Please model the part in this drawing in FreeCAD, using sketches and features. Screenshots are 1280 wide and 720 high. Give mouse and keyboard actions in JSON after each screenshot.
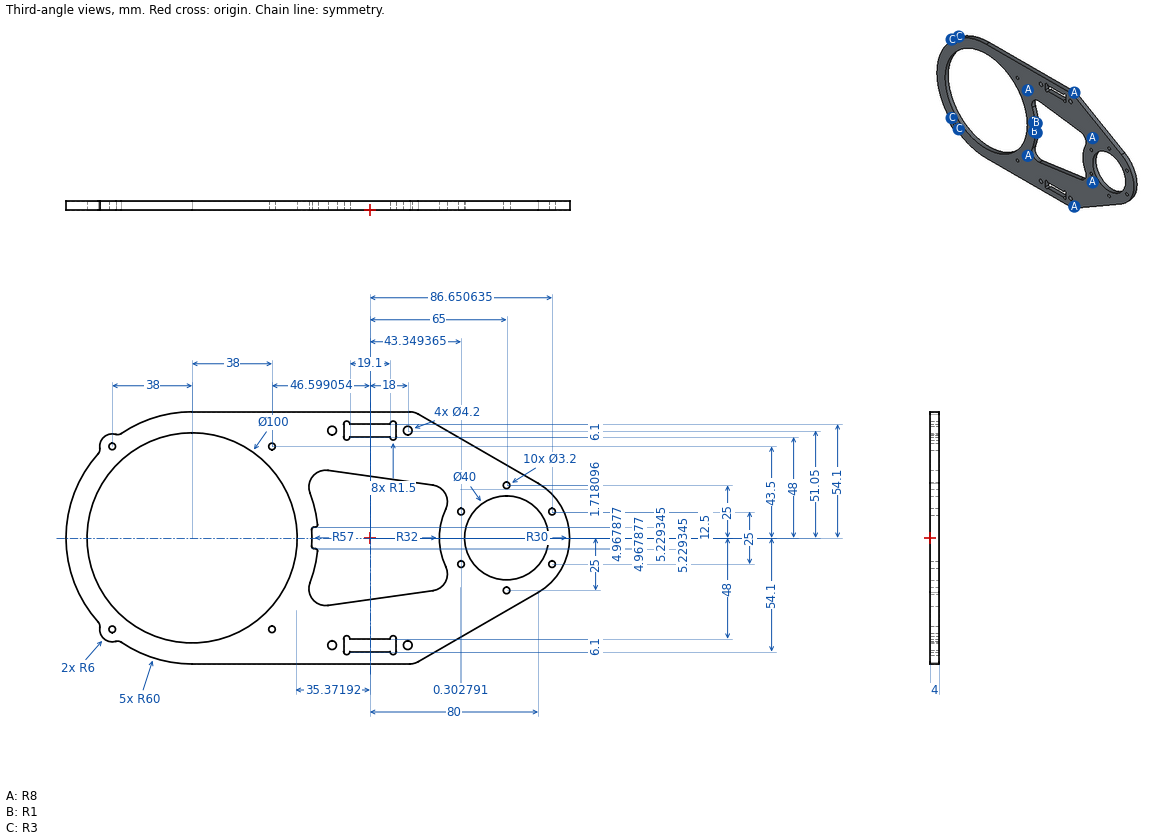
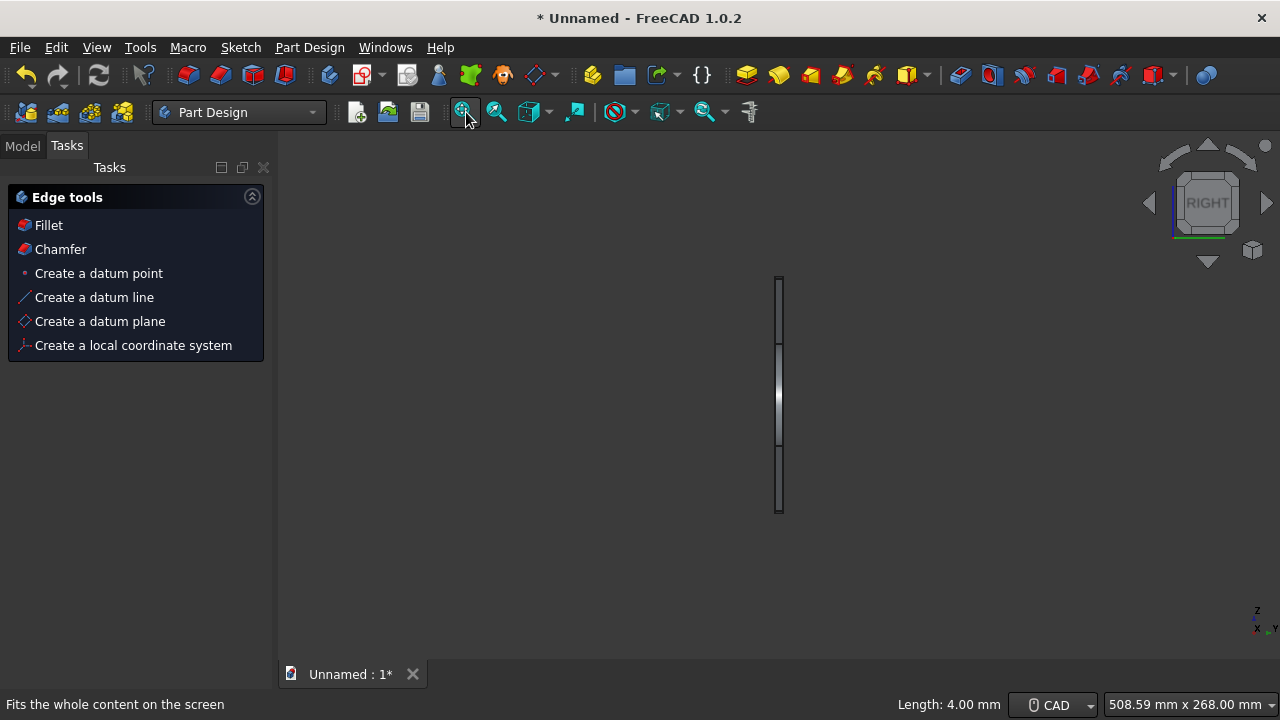
{"action": "key", "text": "5"}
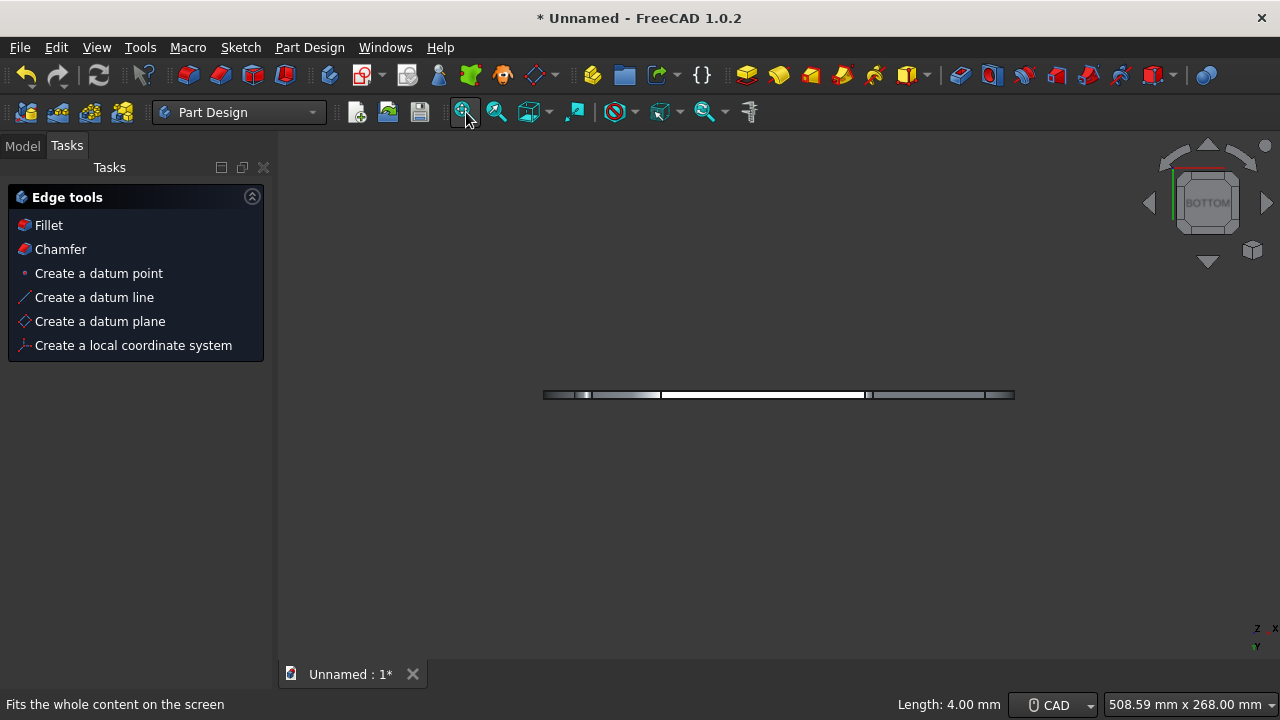
{"action": "scroll", "coordinate": [773, 394], "scroll_direction": "up", "scroll_amount": 9}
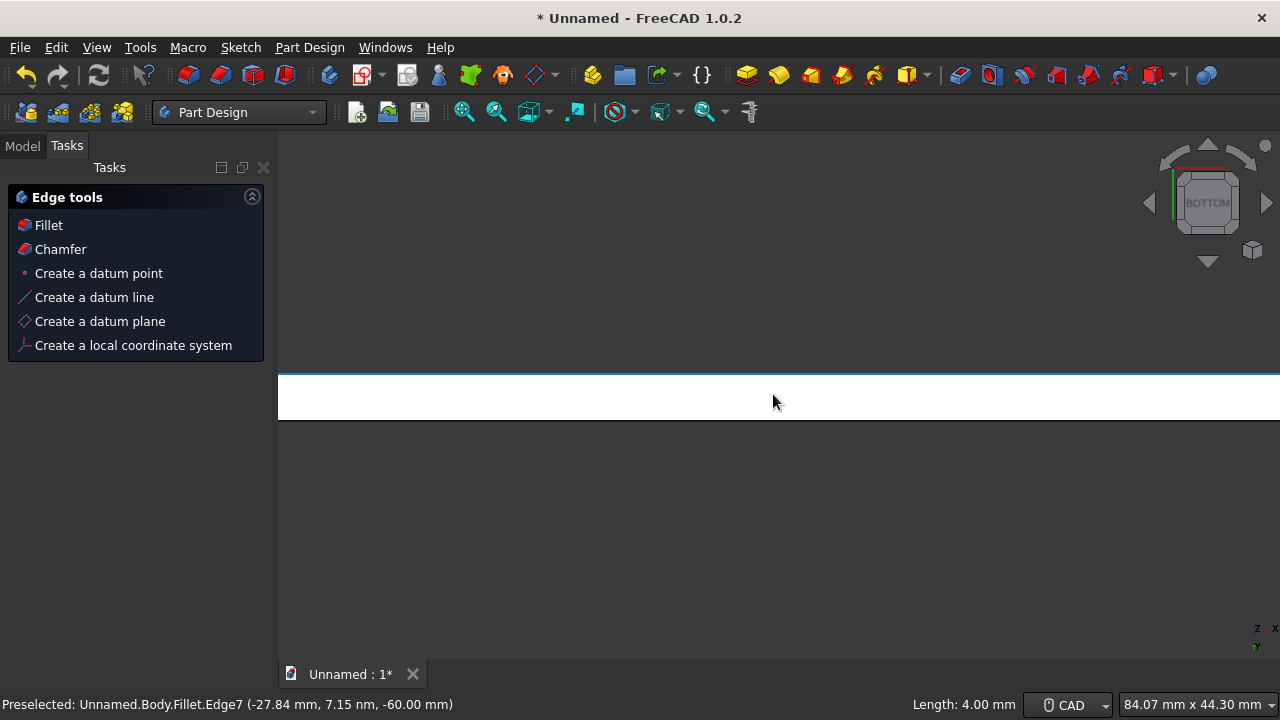
{"action": "left_click", "coordinate": [466, 112]}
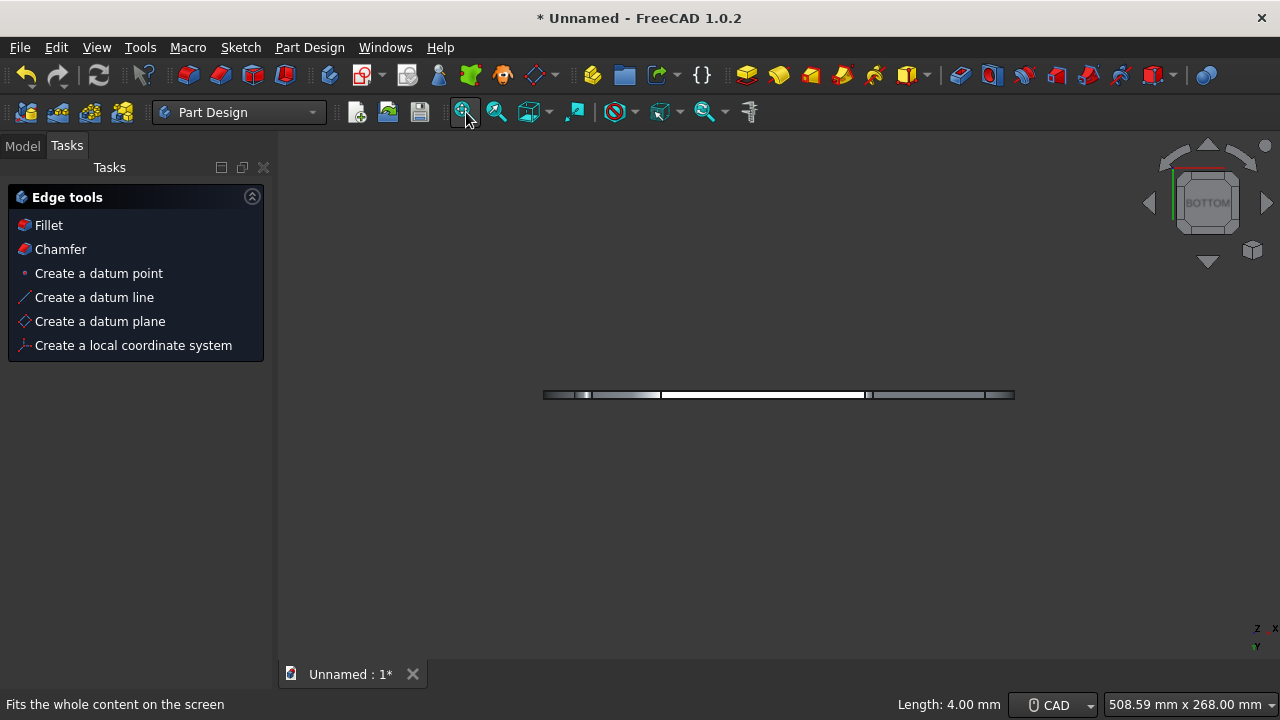
{"action": "key", "text": "4"}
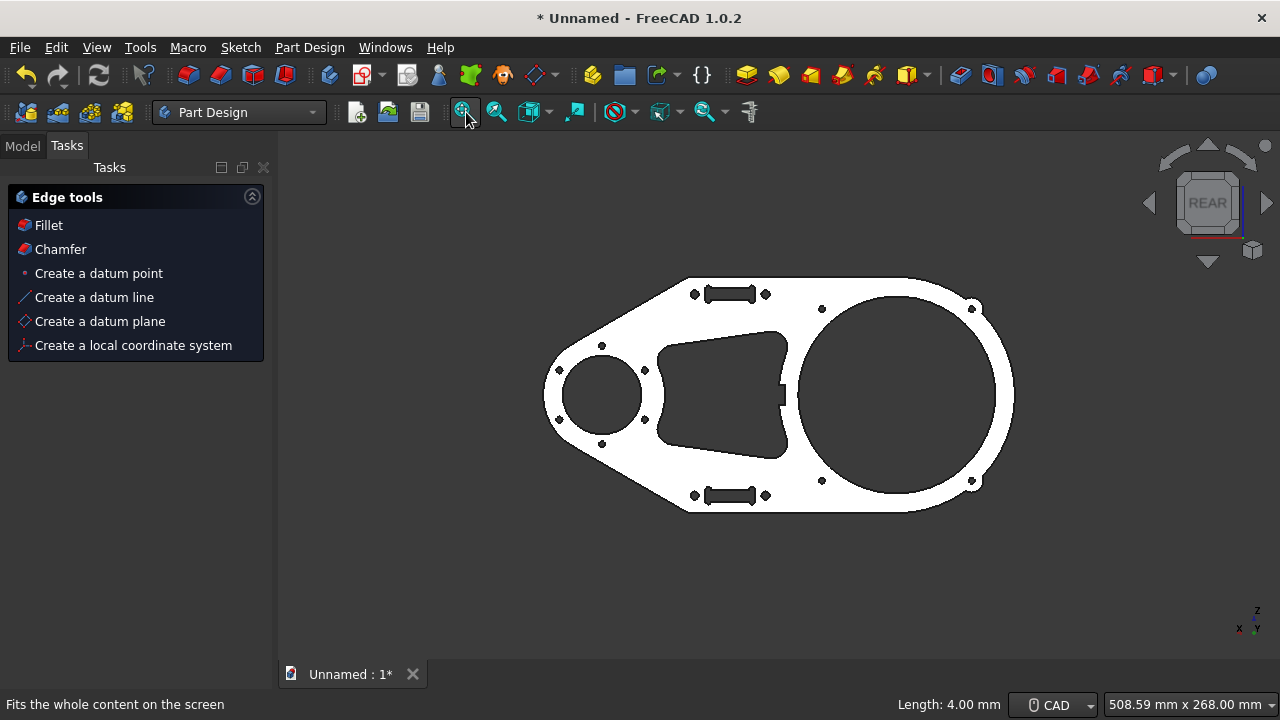
{"action": "scroll", "coordinate": [785, 404], "scroll_direction": "up", "scroll_amount": 9}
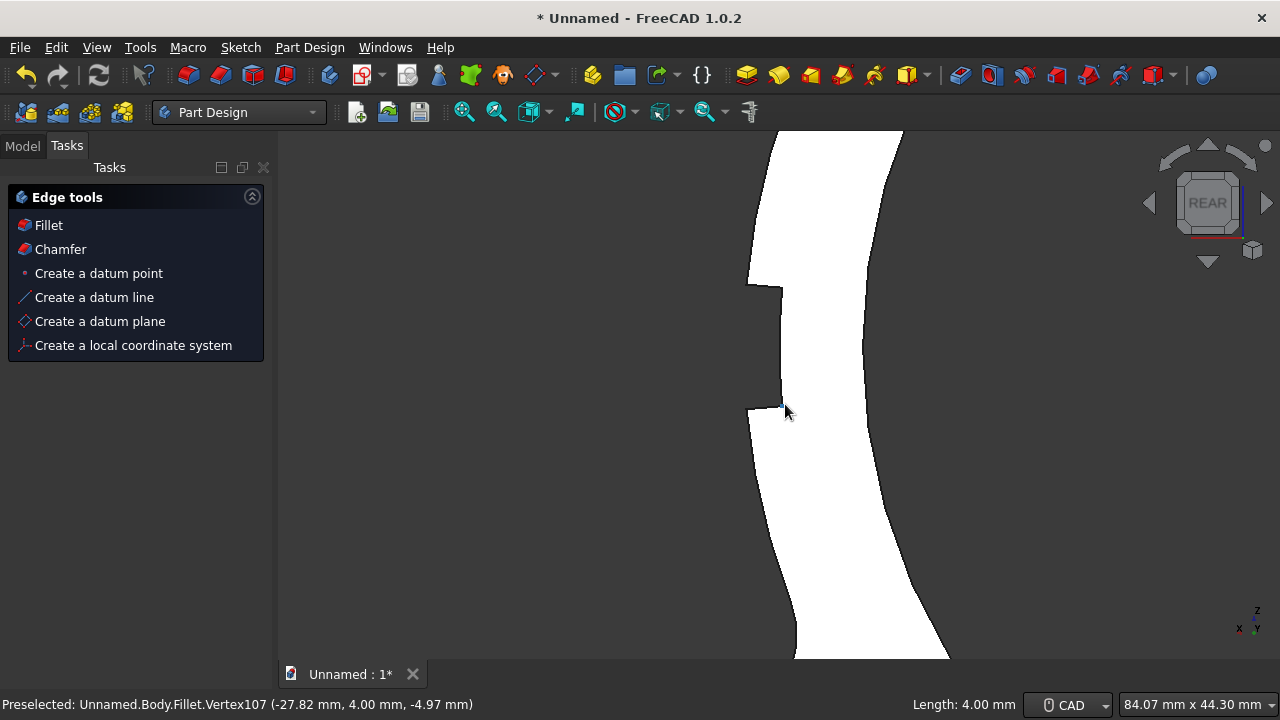
{"action": "key", "text": "v f"}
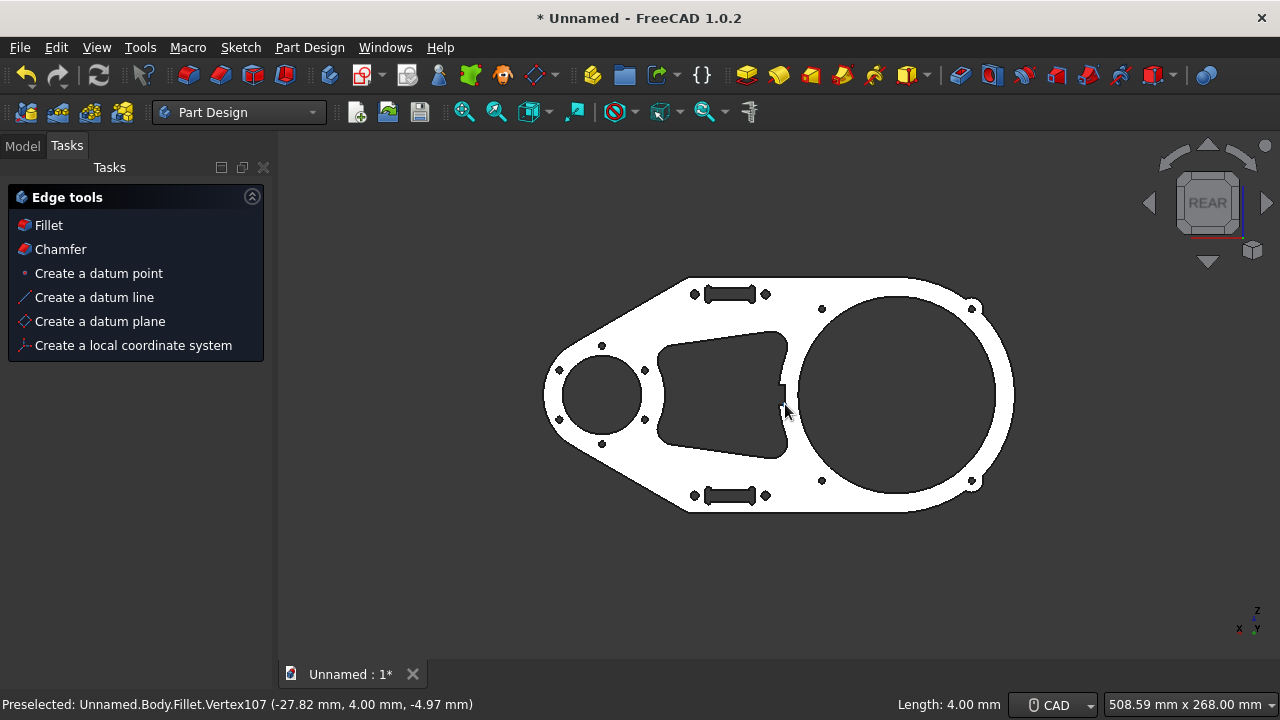
{"action": "key", "text": "6"}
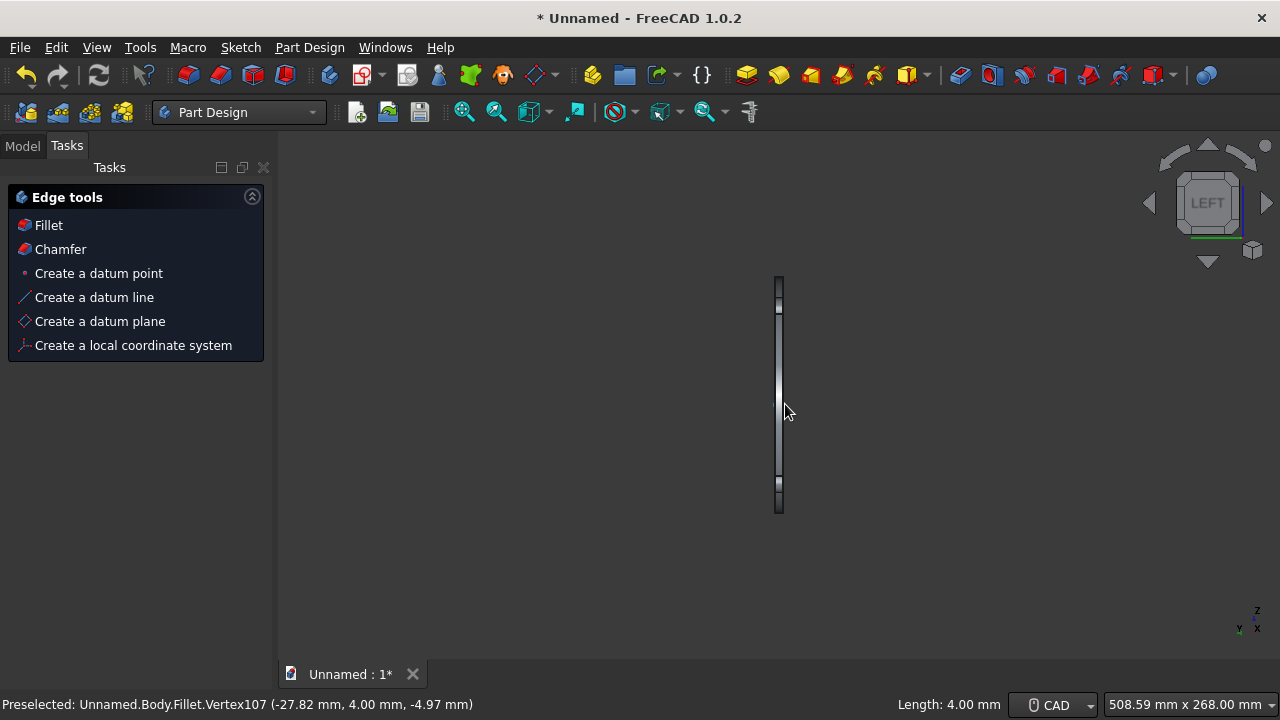
{"action": "left_click", "coordinate": [466, 112]}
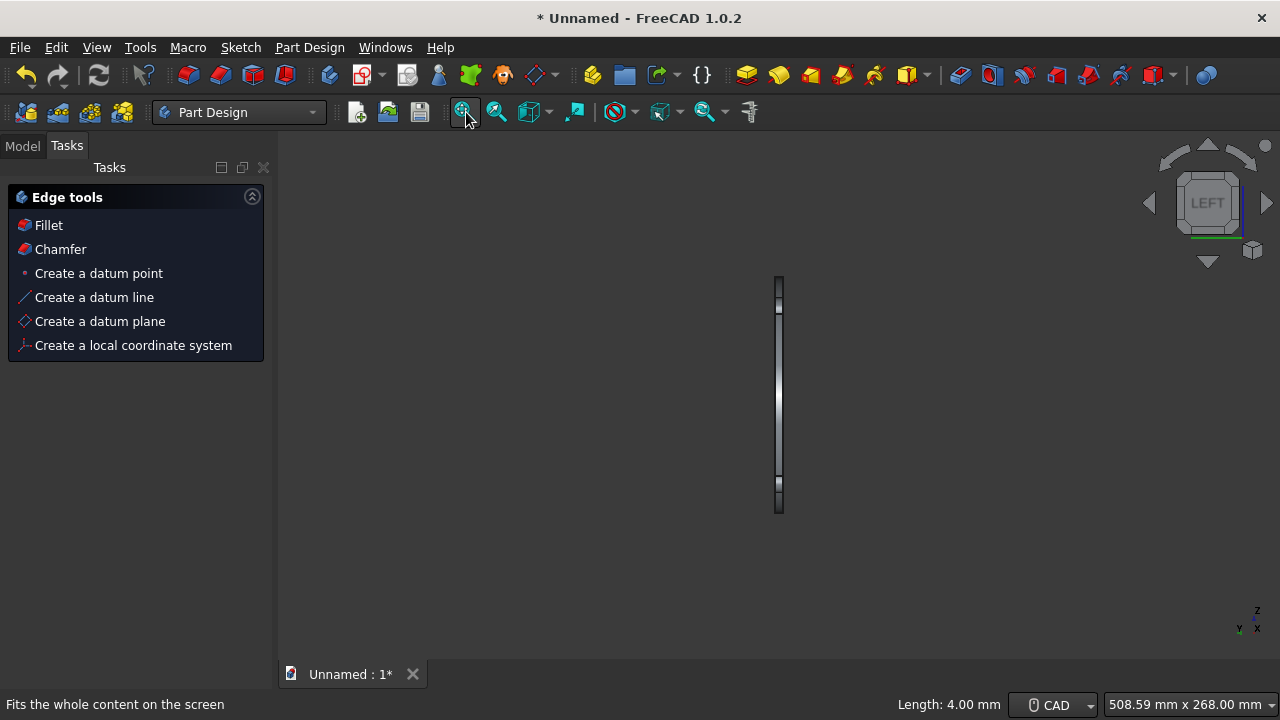
{"action": "scroll", "coordinate": [779, 404], "scroll_direction": "up", "scroll_amount": 9}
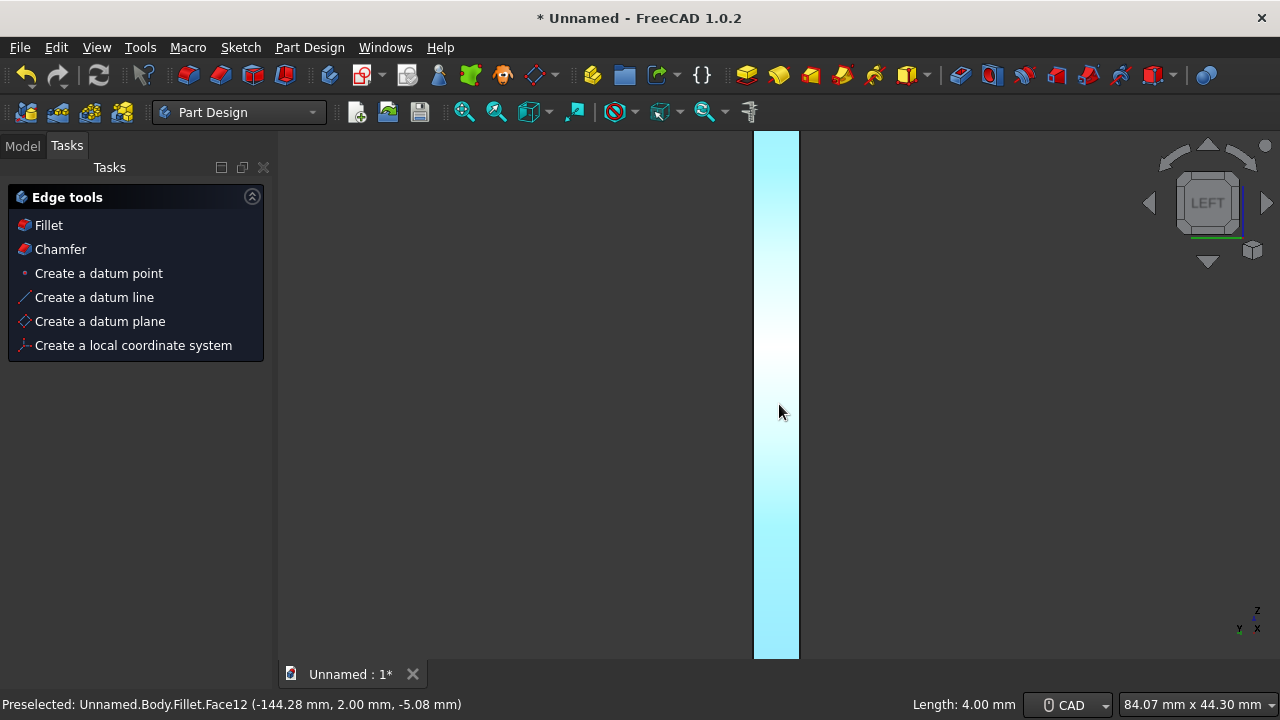
{"action": "left_click", "coordinate": [466, 112]}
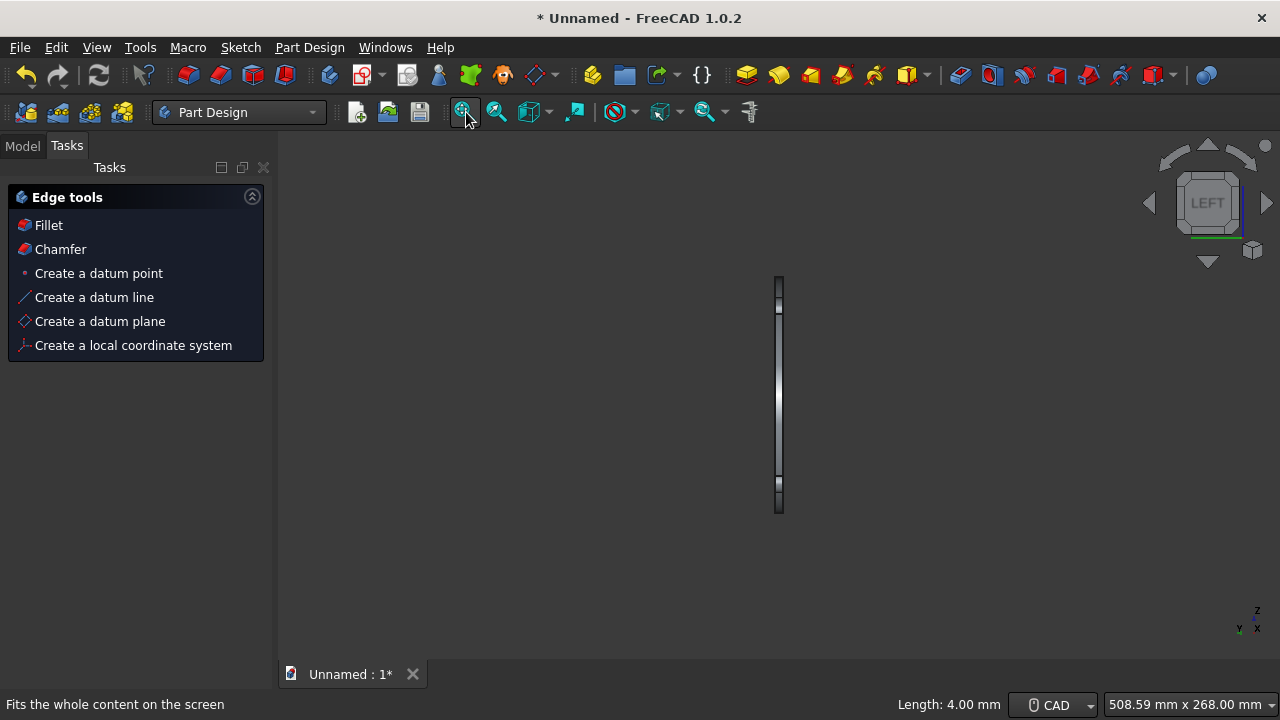
{"action": "key", "text": "v 3"}